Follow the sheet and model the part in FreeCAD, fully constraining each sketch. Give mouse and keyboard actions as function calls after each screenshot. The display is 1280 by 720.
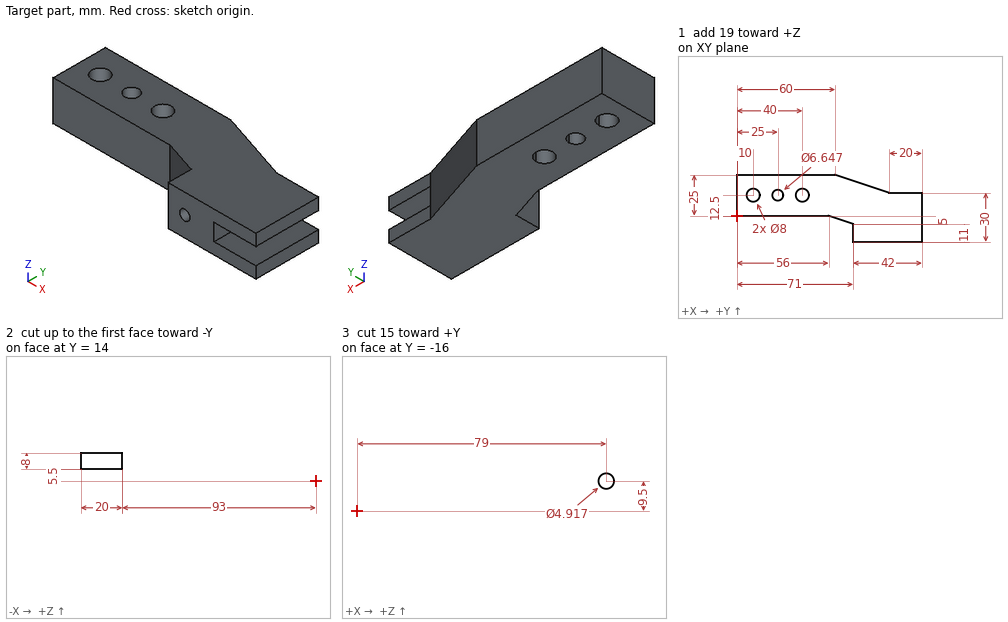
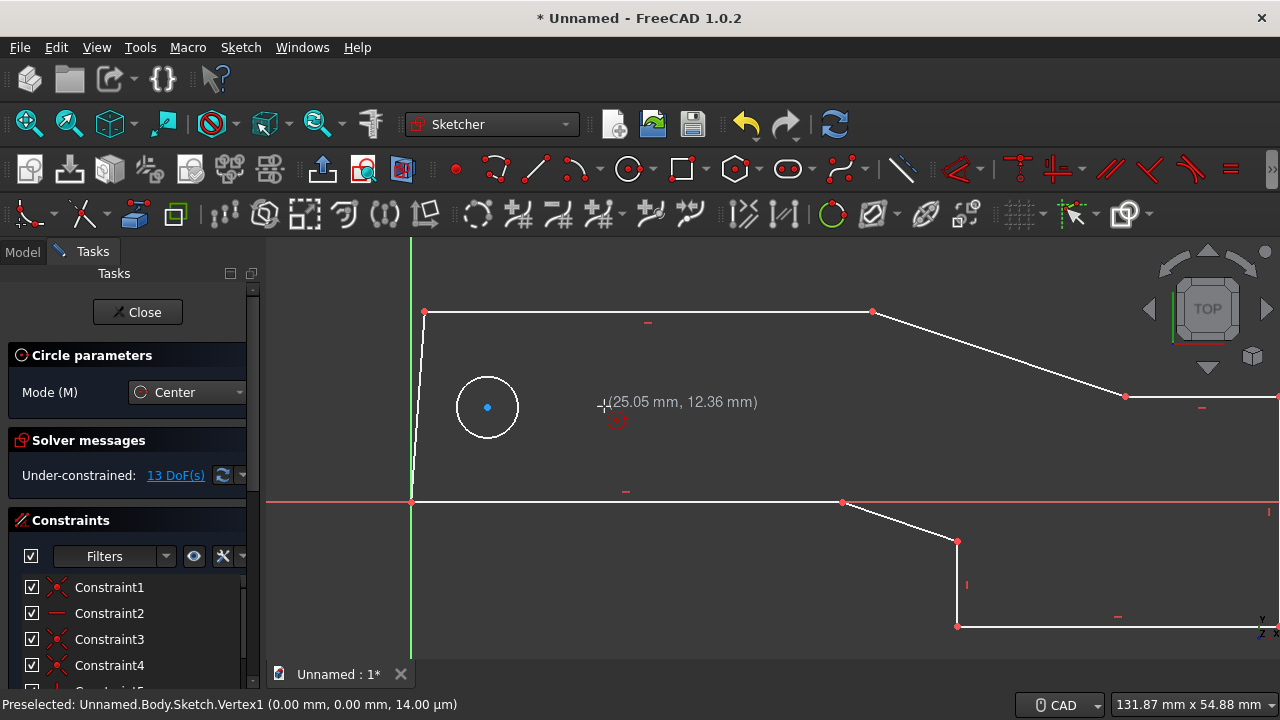
click(603, 406)
click(621, 388)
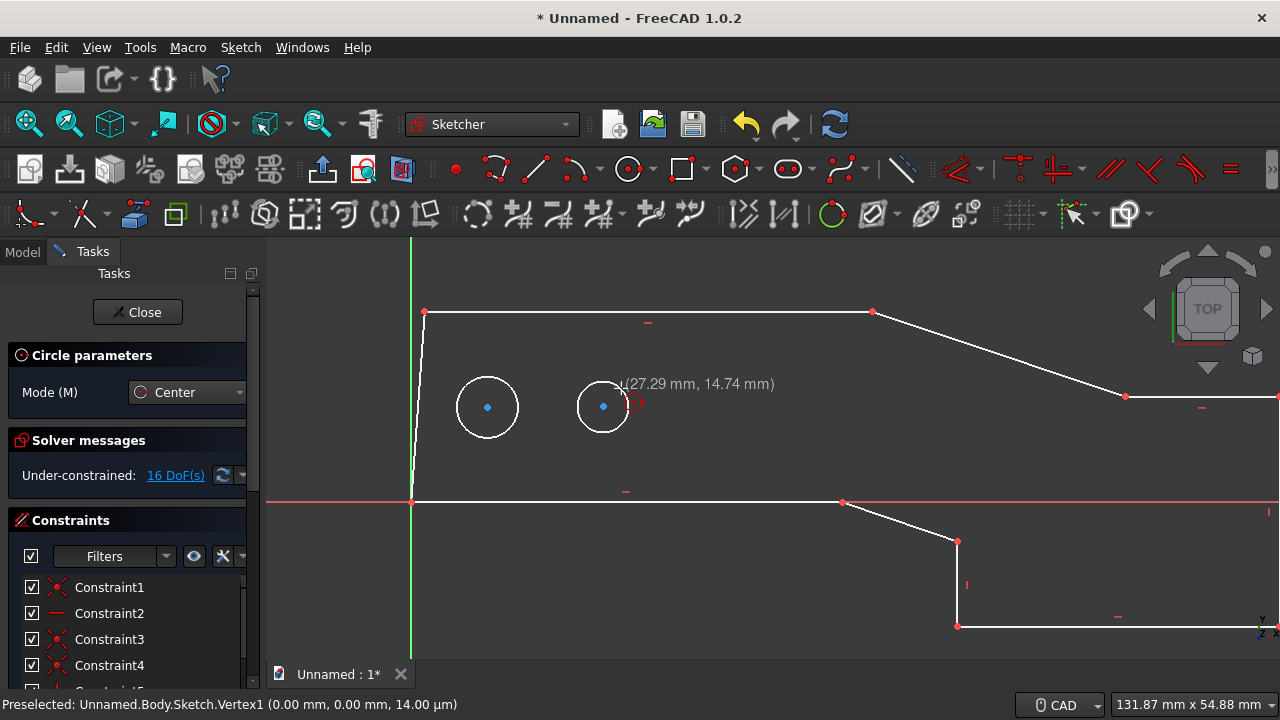
click(719, 406)
click(741, 384)
key(Escape)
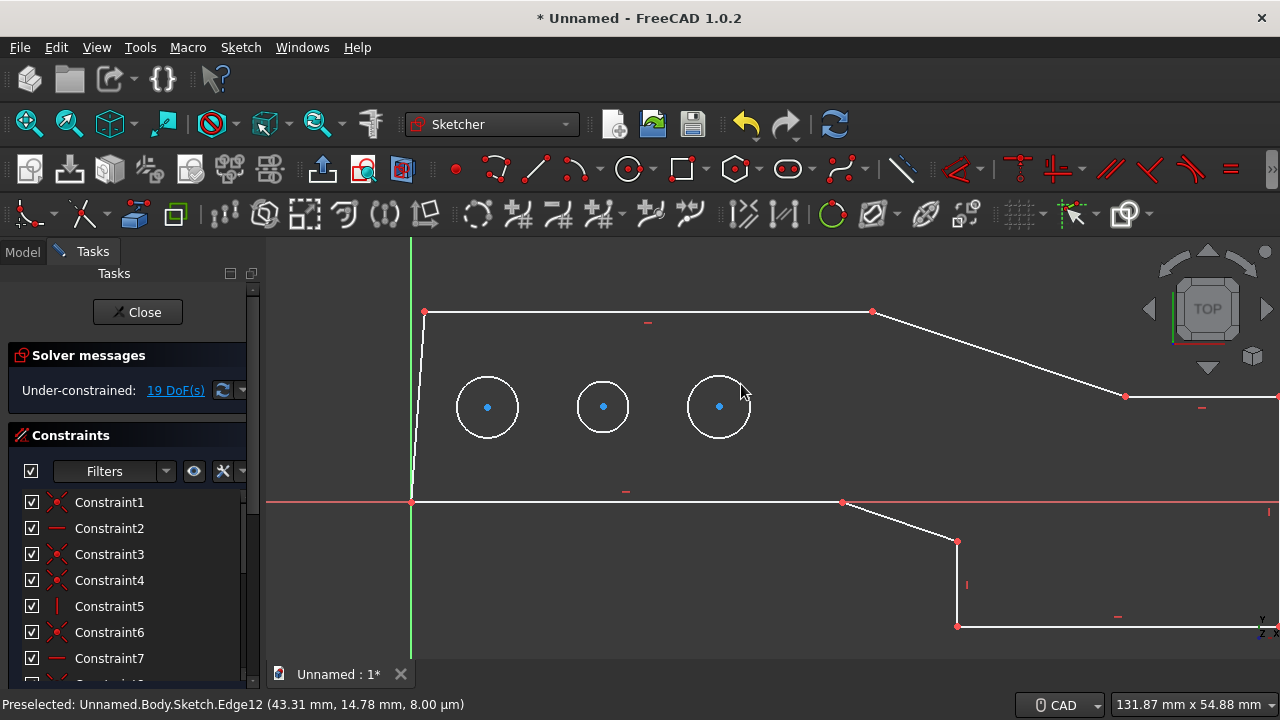
scroll(421, 369, up, 2)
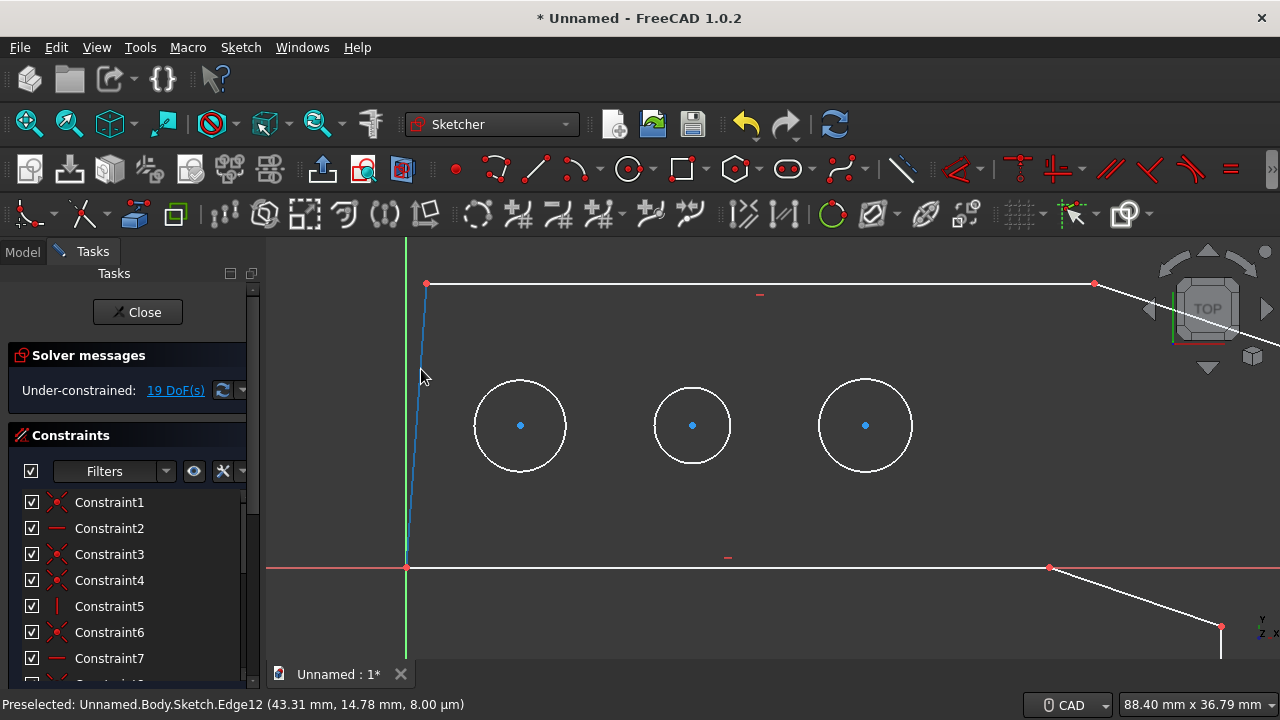
click(421, 369)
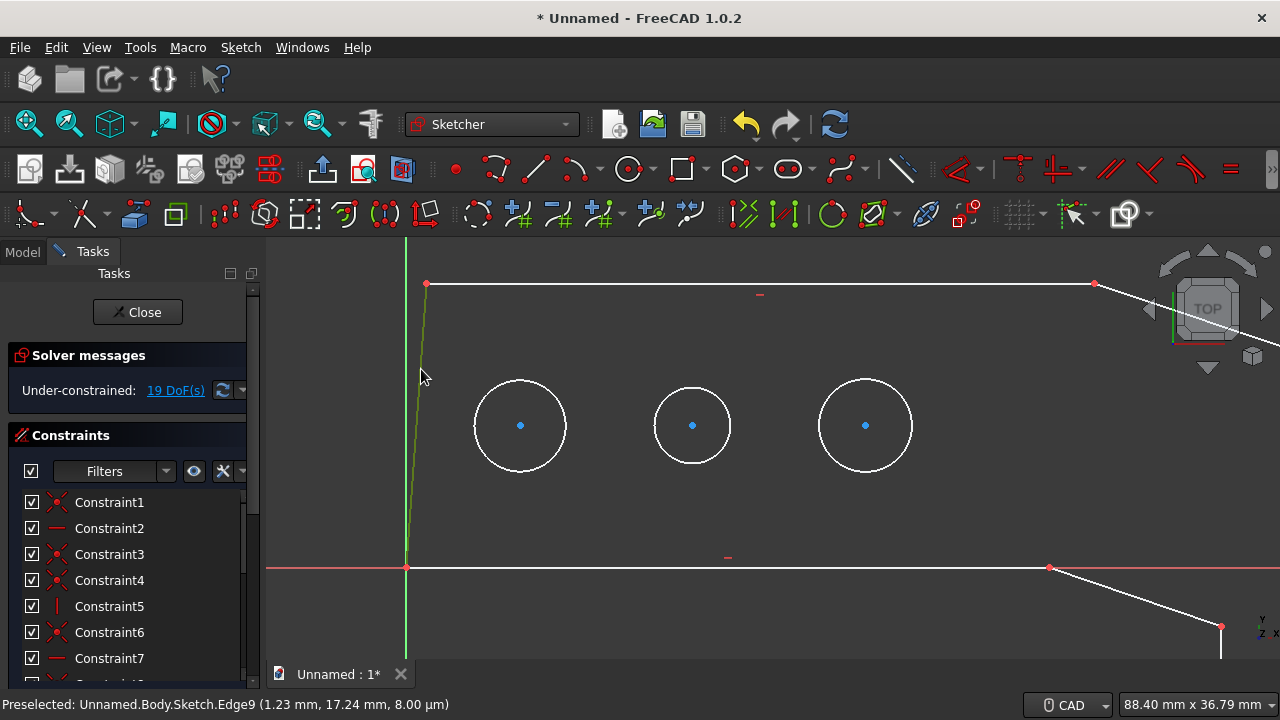
key(v)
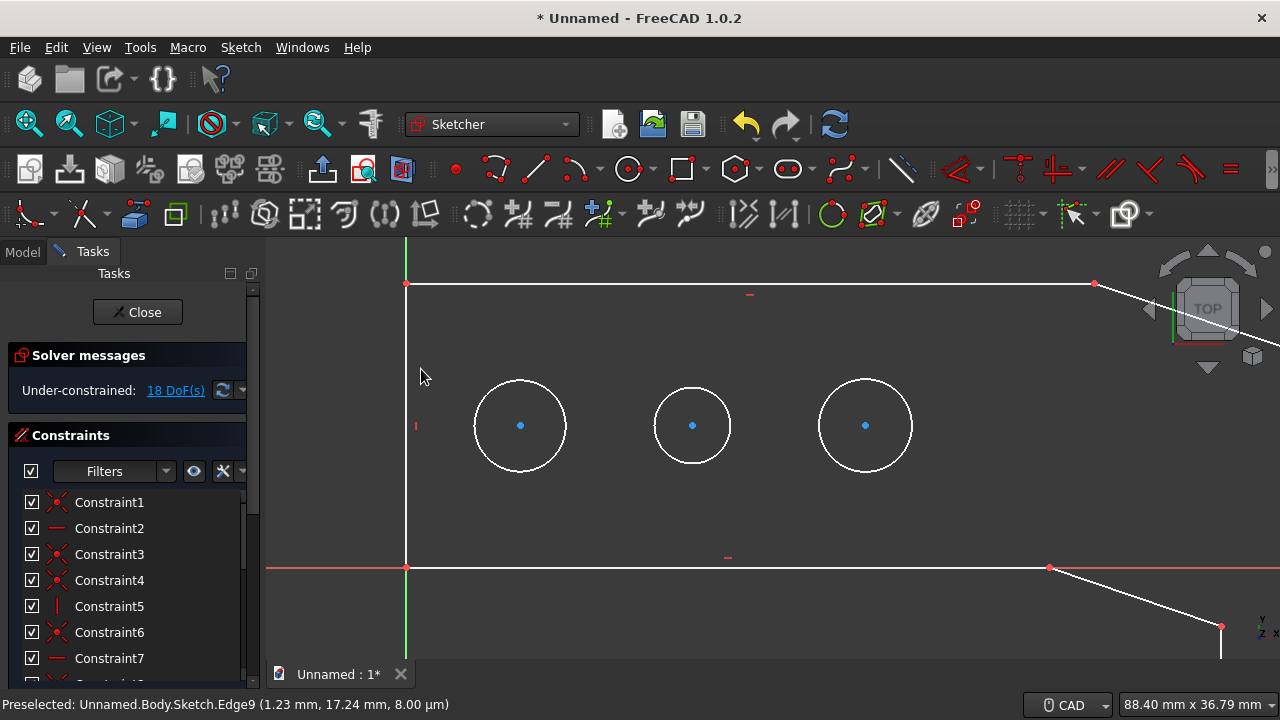
click(552, 394)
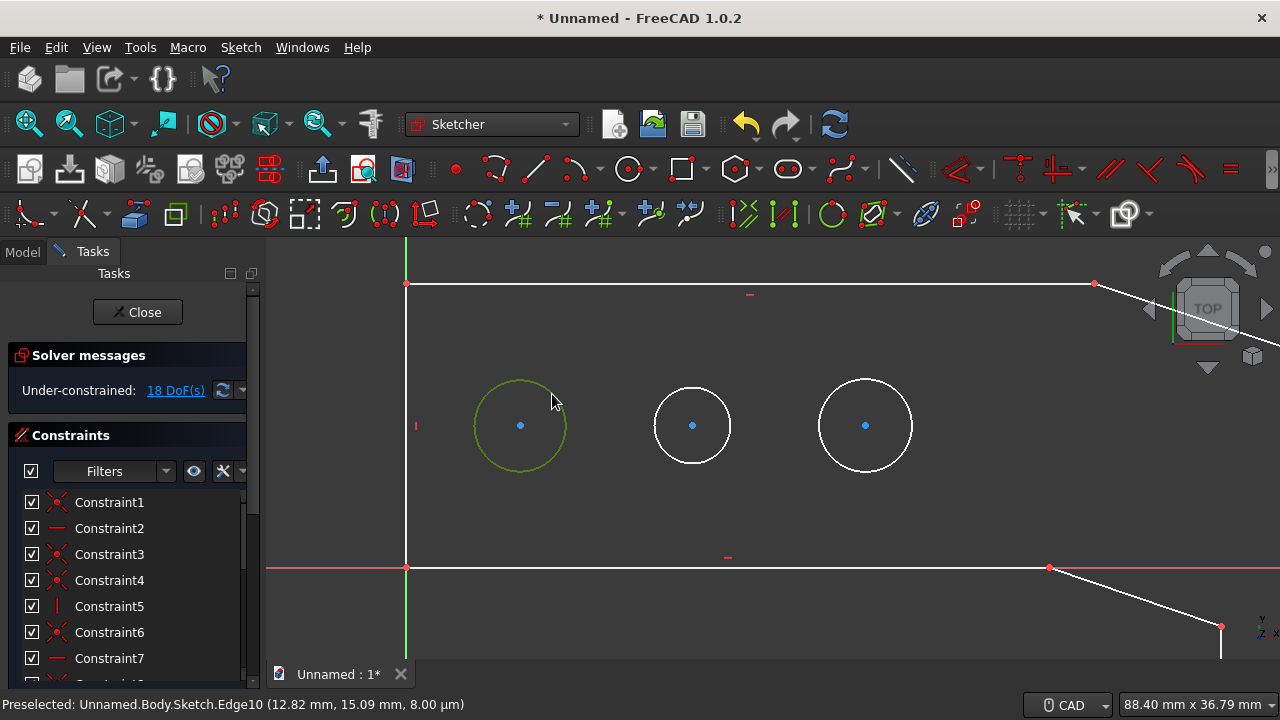
click(898, 393)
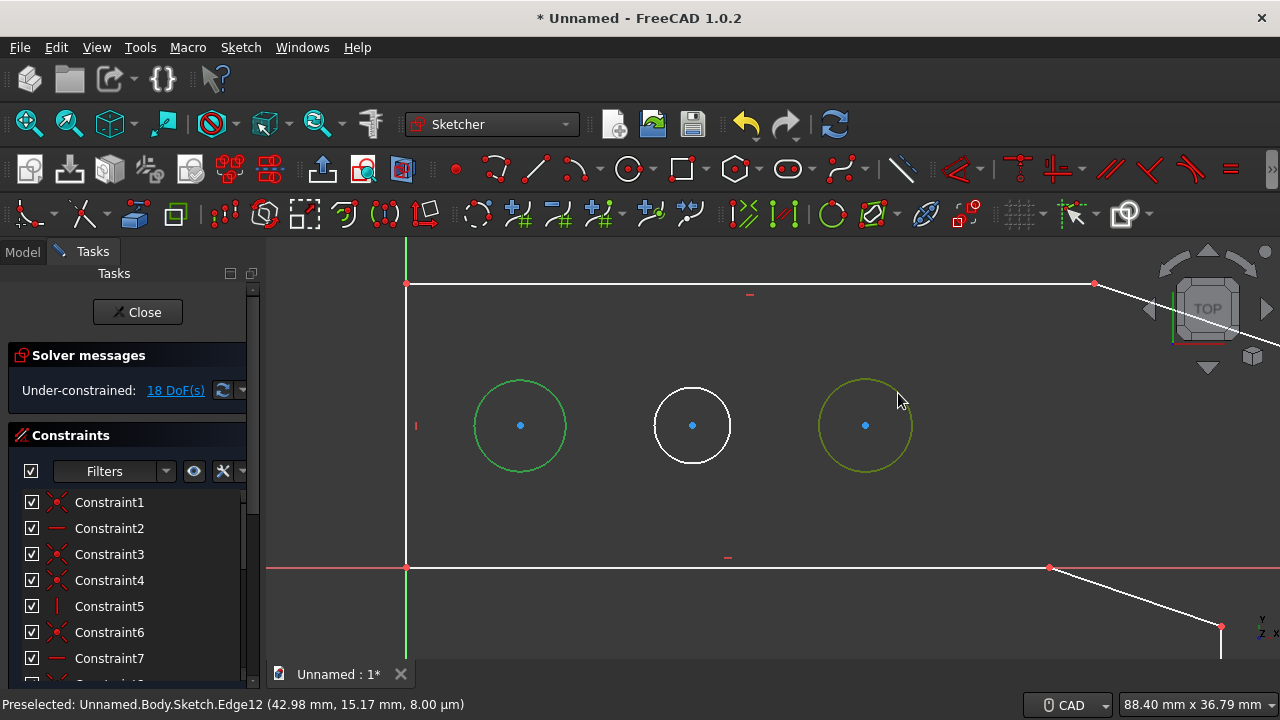
click(1232, 170)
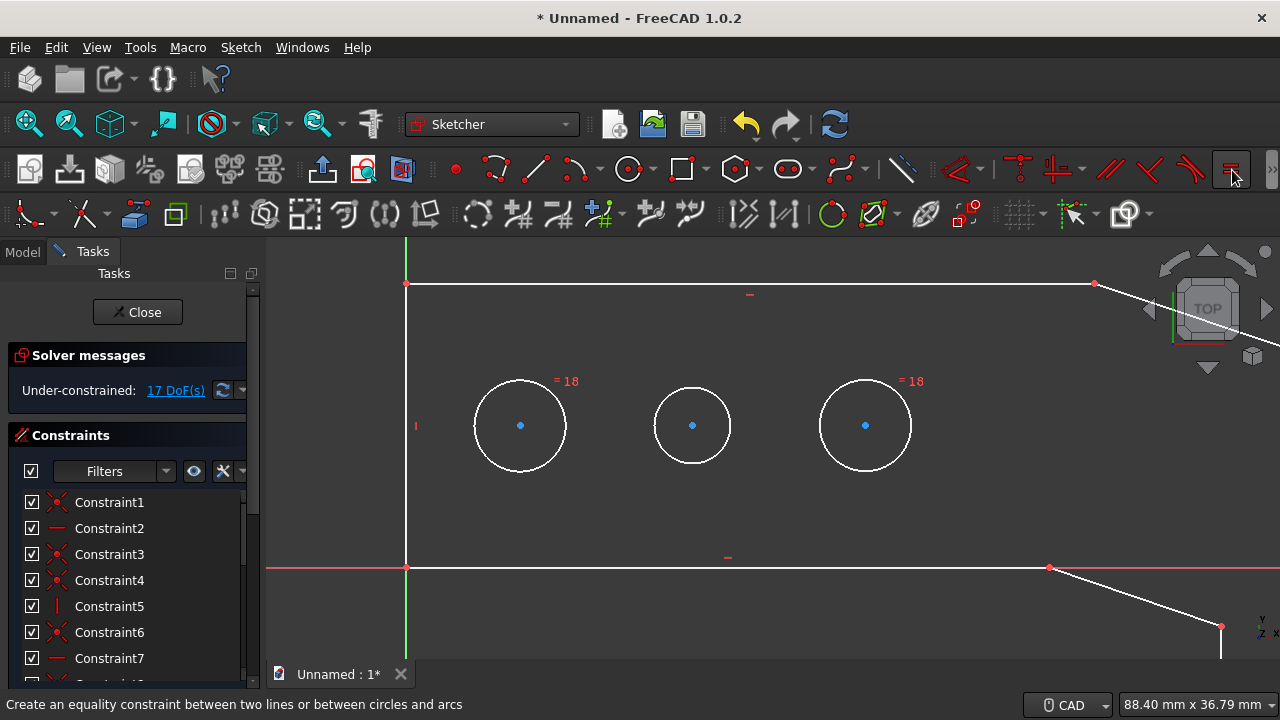
click(520, 426)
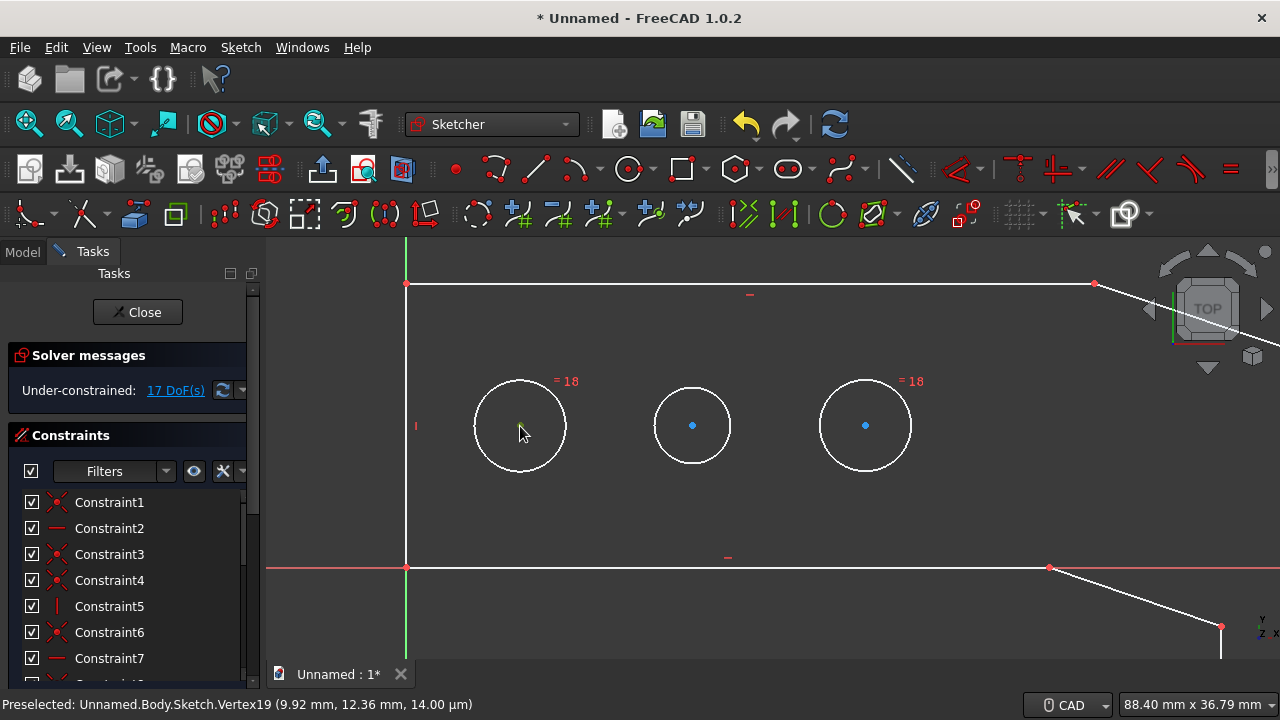
click(692, 426)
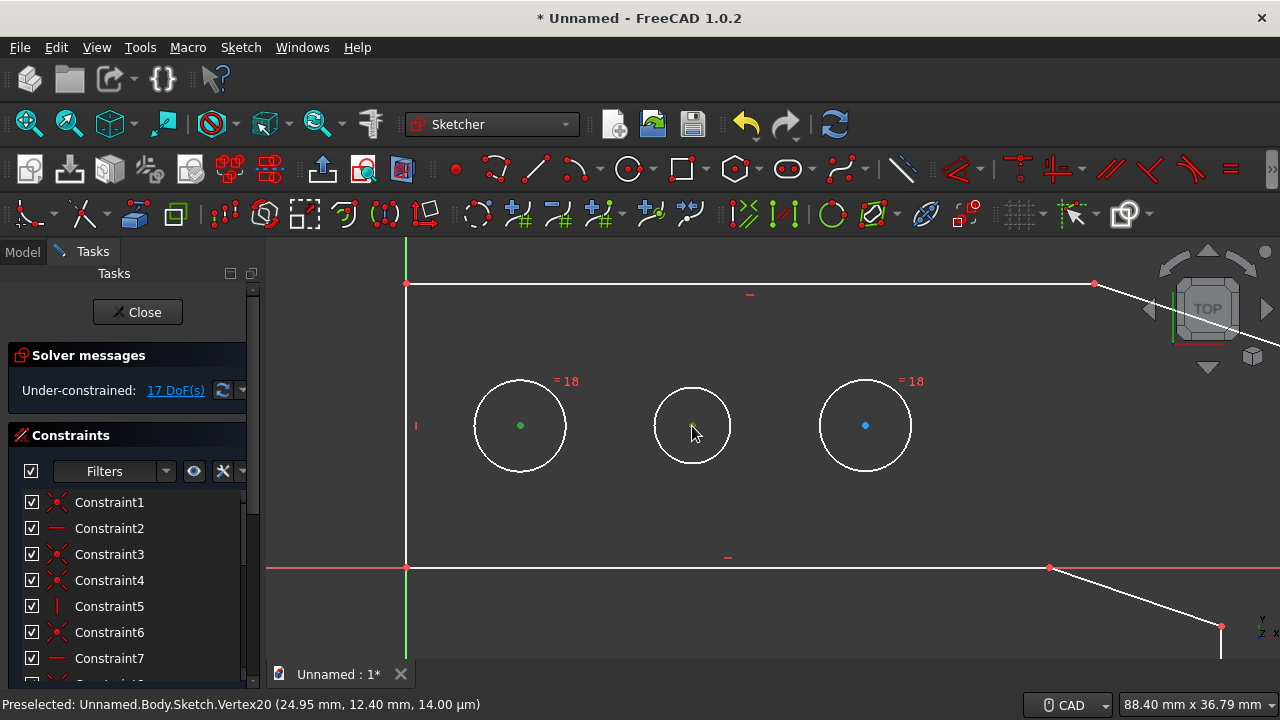
click(1084, 170)